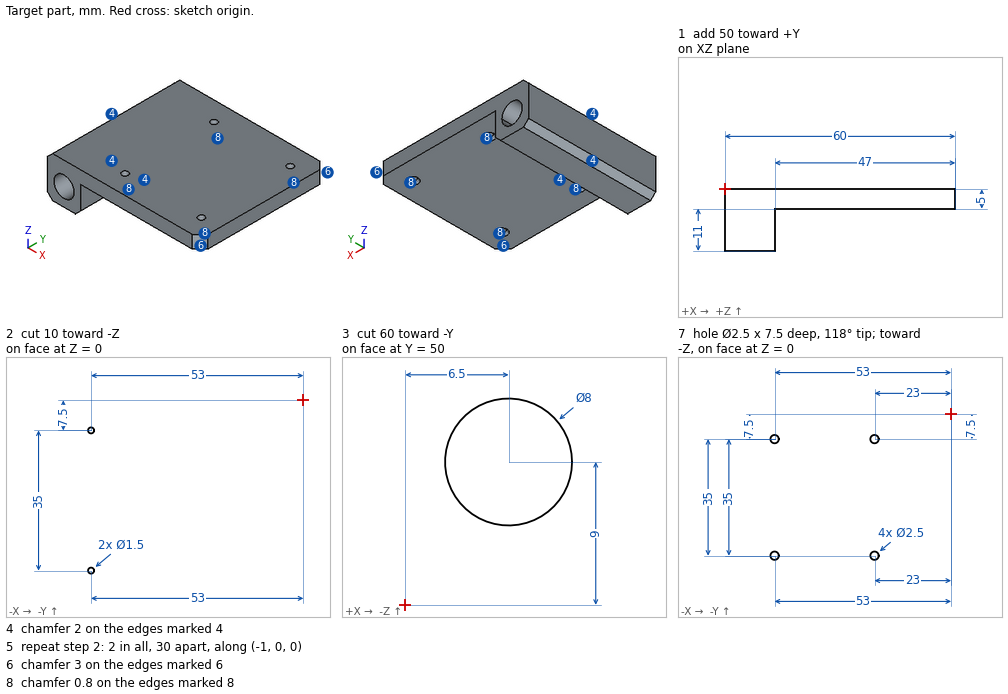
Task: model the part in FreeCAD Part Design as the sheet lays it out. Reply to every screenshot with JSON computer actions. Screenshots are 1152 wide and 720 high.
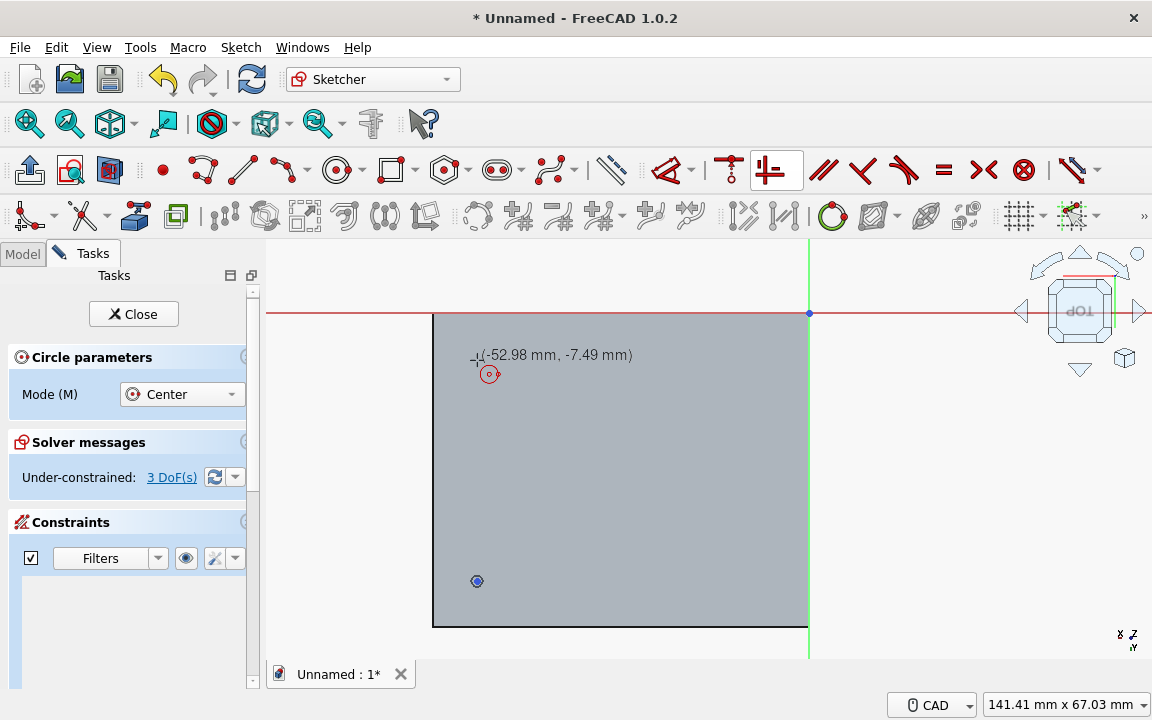
{"action": "left_click", "coordinate": [477, 360]}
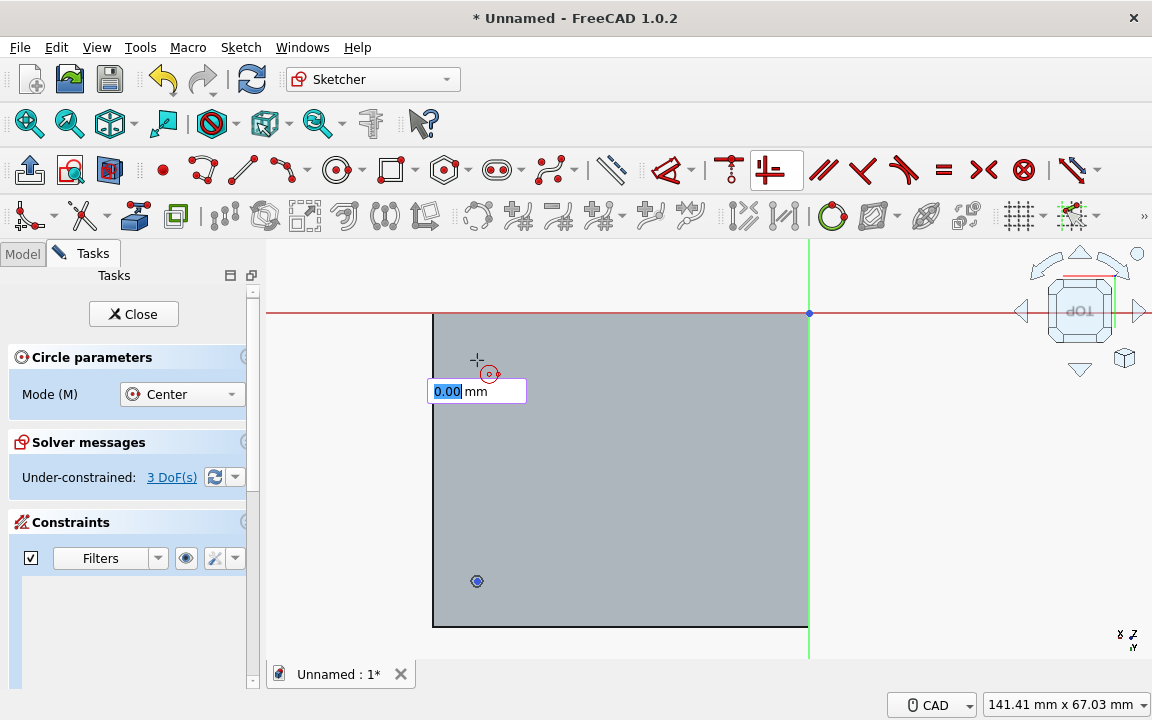
{"action": "scroll", "coordinate": [480, 357], "scroll_direction": "up", "scroll_amount": 7}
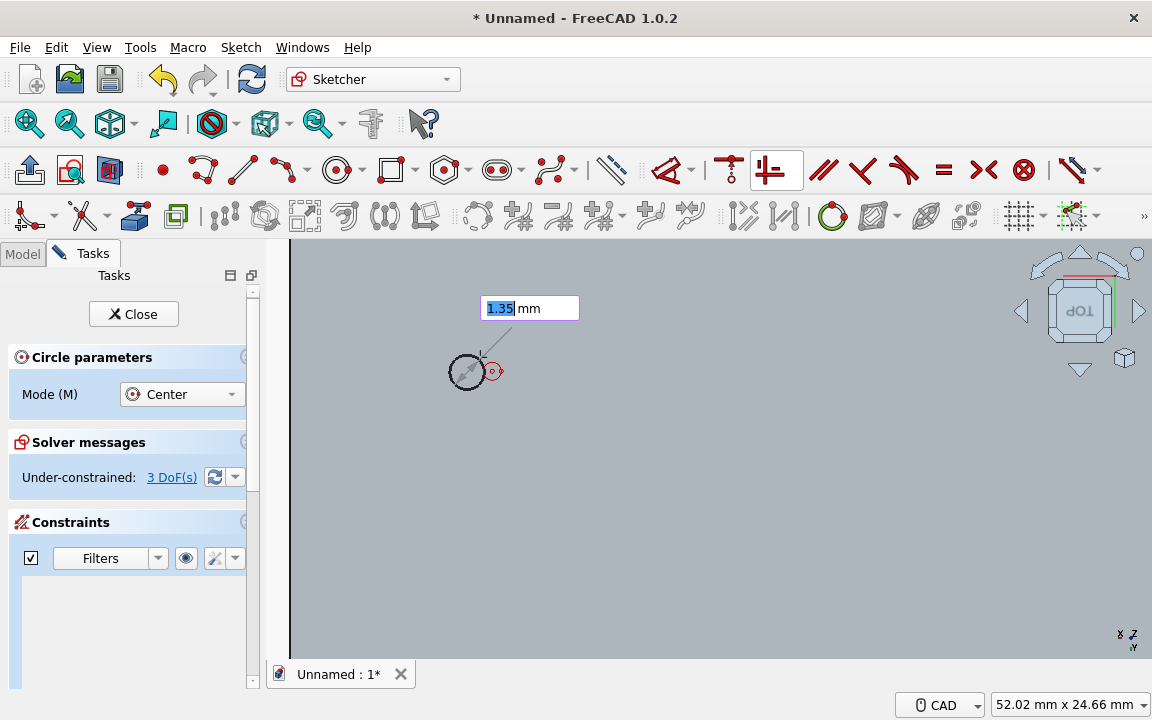
{"action": "left_click", "coordinate": [481, 357]}
{"action": "key", "text": "Escape"}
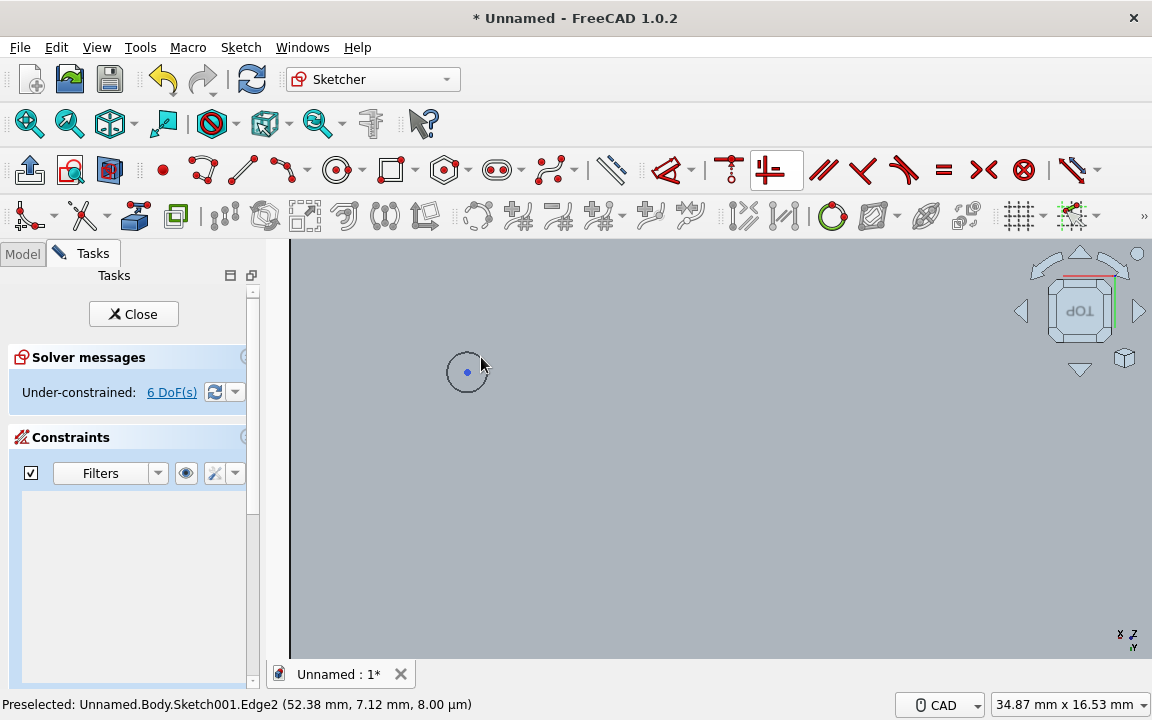
{"action": "scroll", "coordinate": [480, 357], "scroll_direction": "down", "scroll_amount": 7}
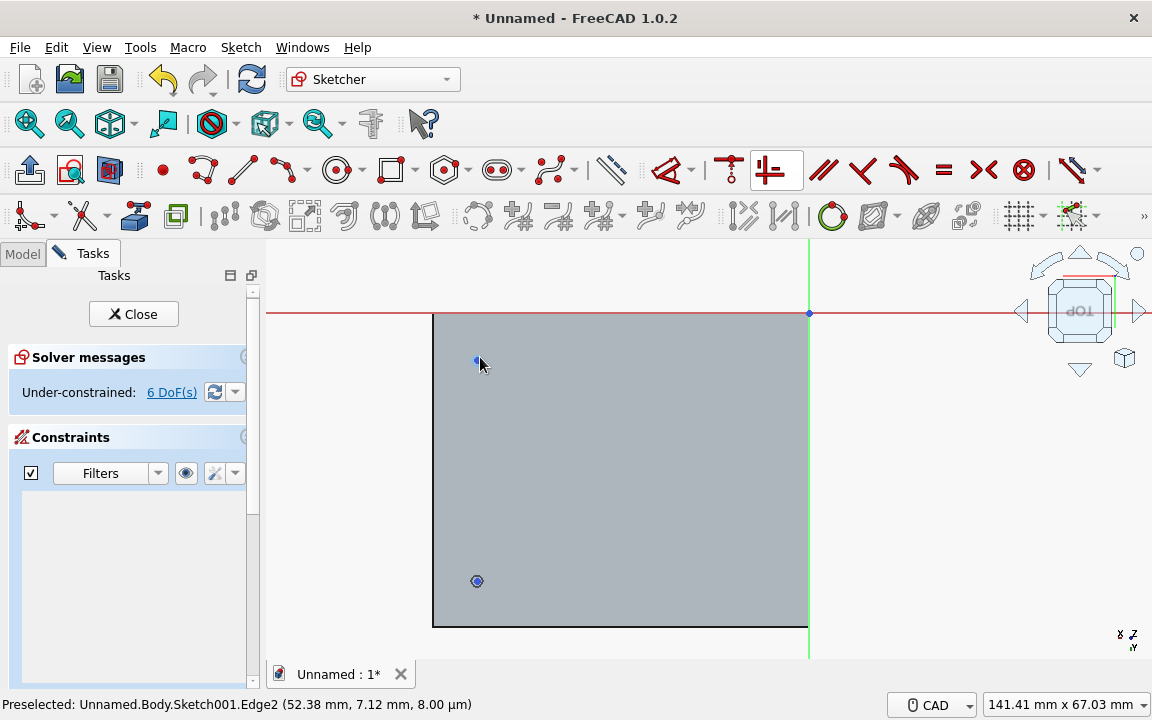
{"action": "scroll", "coordinate": [481, 577], "scroll_direction": "up", "scroll_amount": 5}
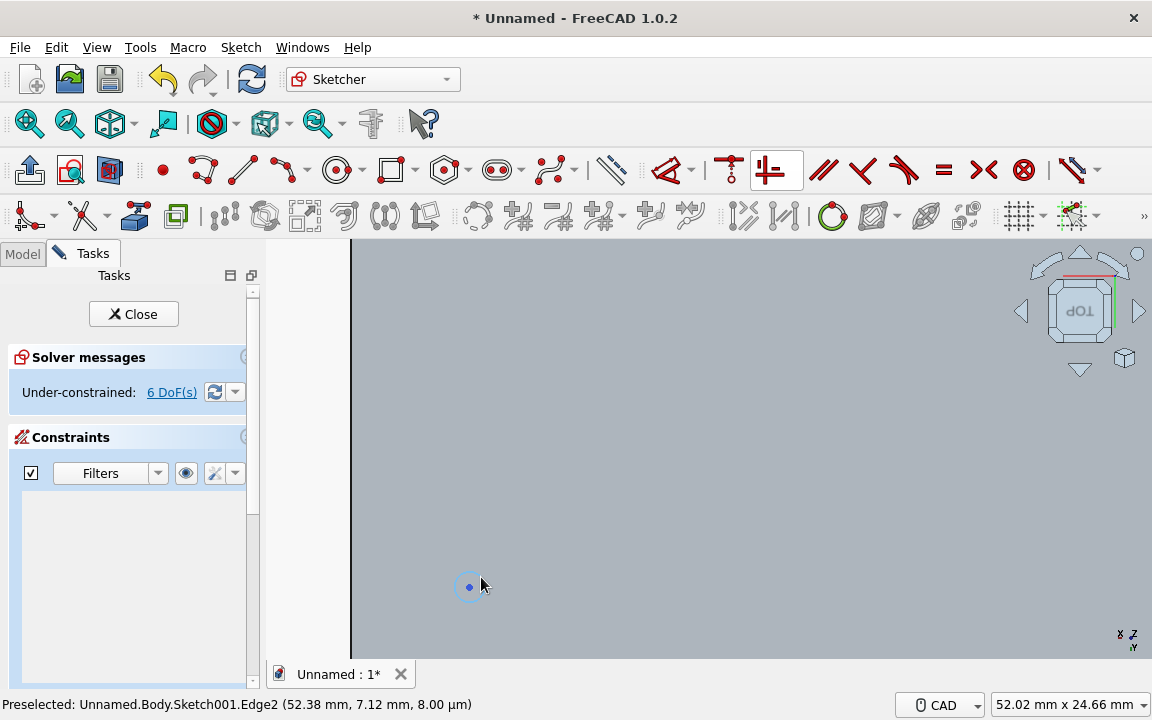
{"action": "left_click", "coordinate": [480, 576]}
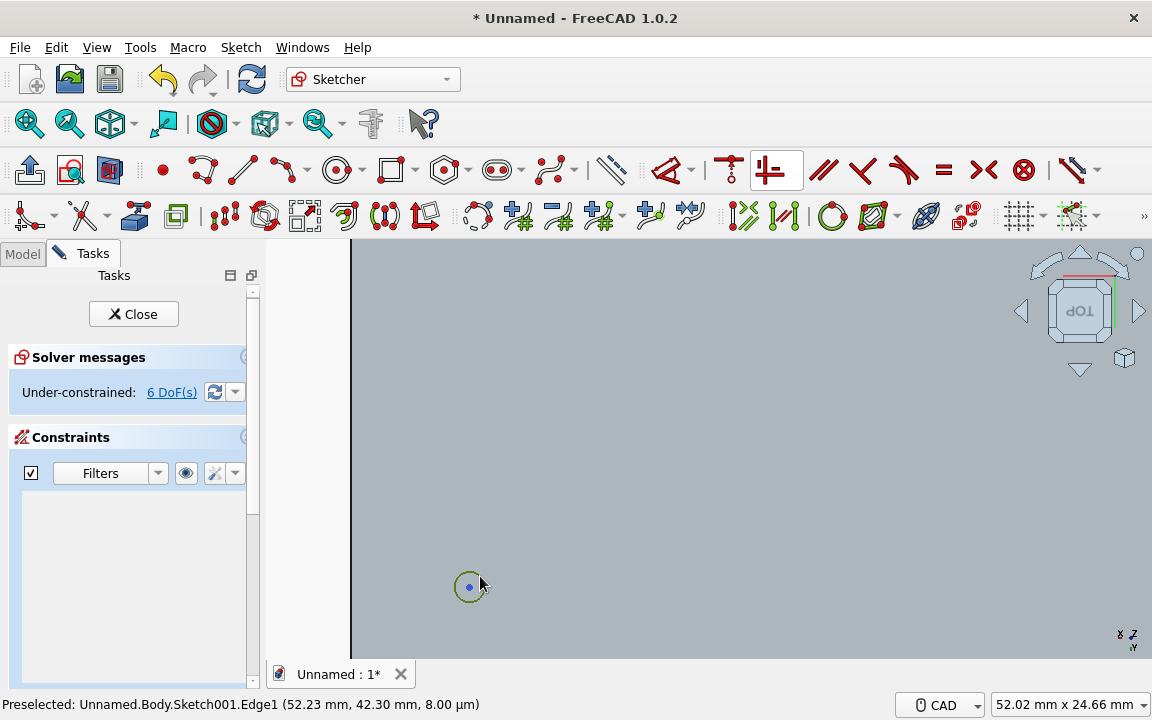
{"action": "scroll", "coordinate": [481, 578], "scroll_direction": "down", "scroll_amount": 5}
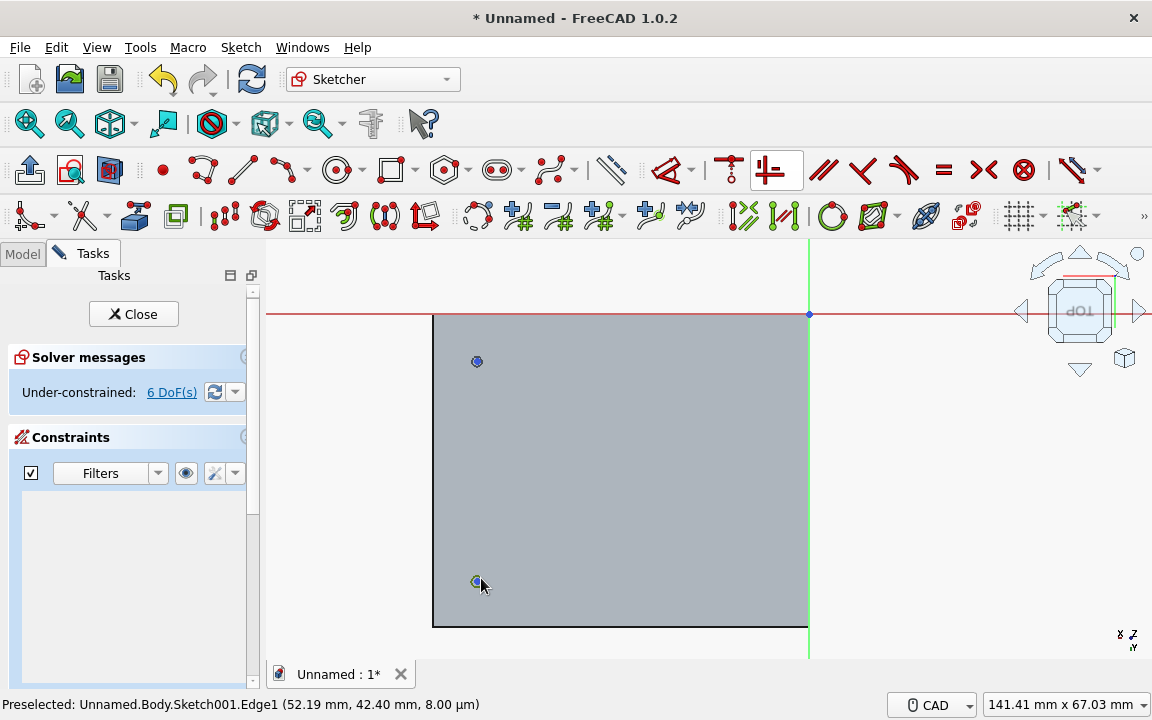
{"action": "scroll", "coordinate": [480, 358], "scroll_direction": "up", "scroll_amount": 6}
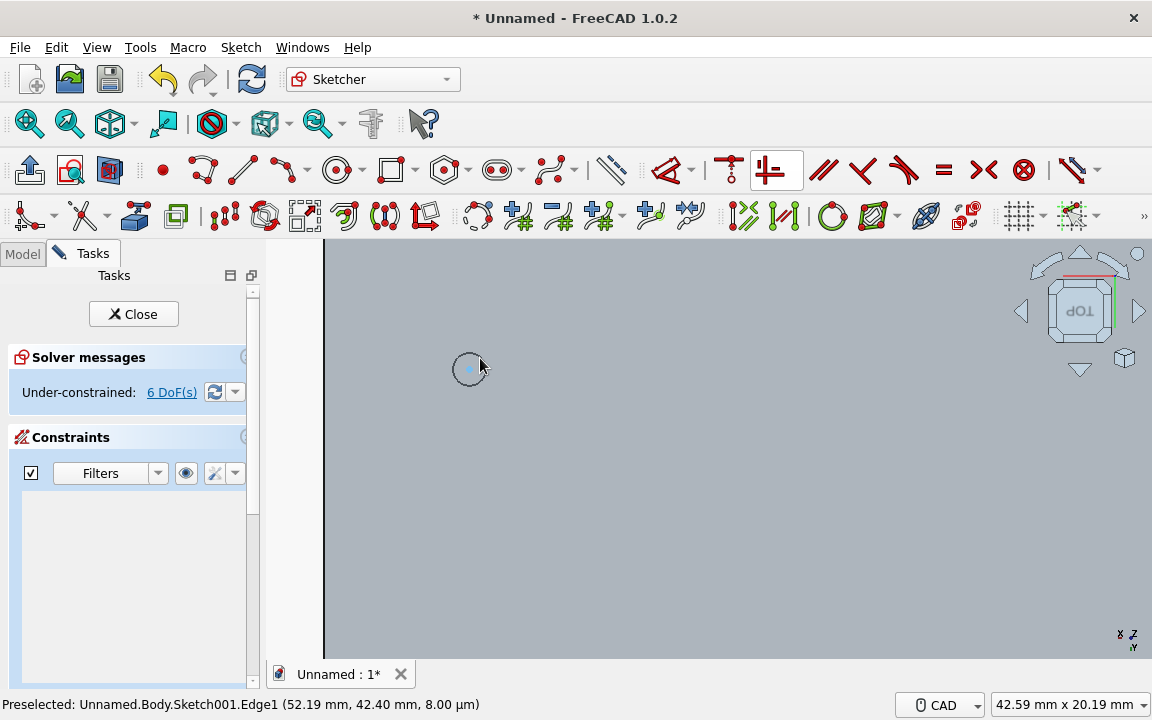
{"action": "left_click", "coordinate": [481, 358]}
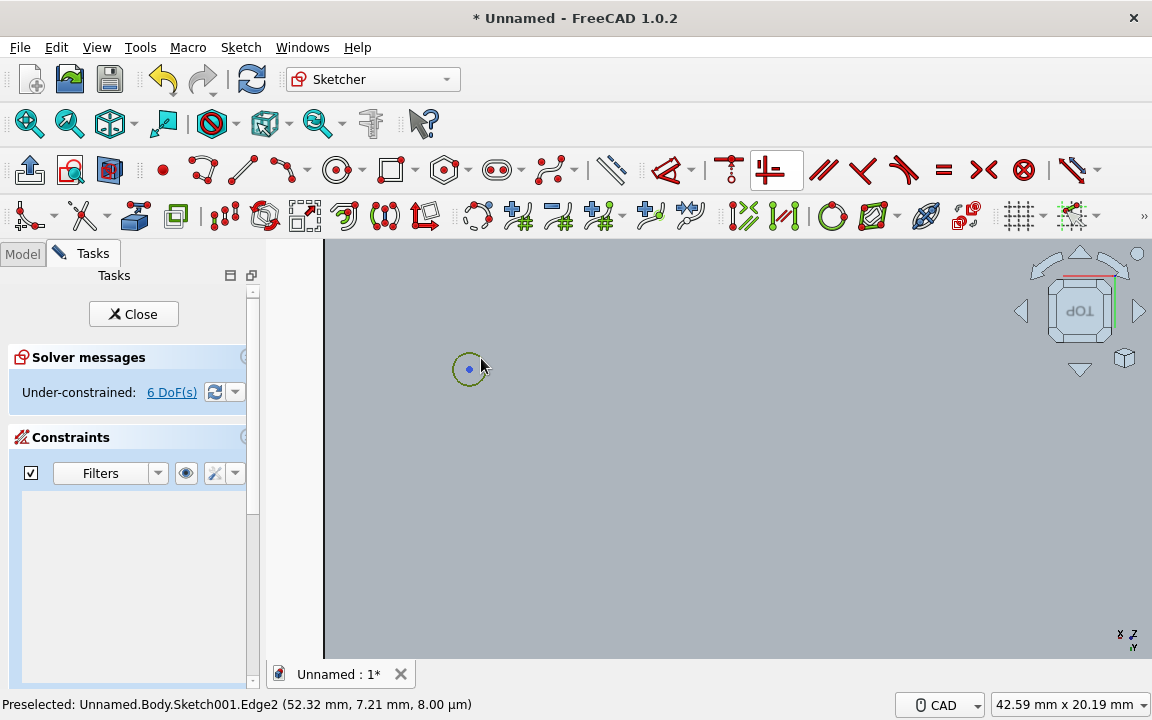
{"action": "left_click", "coordinate": [944, 170]}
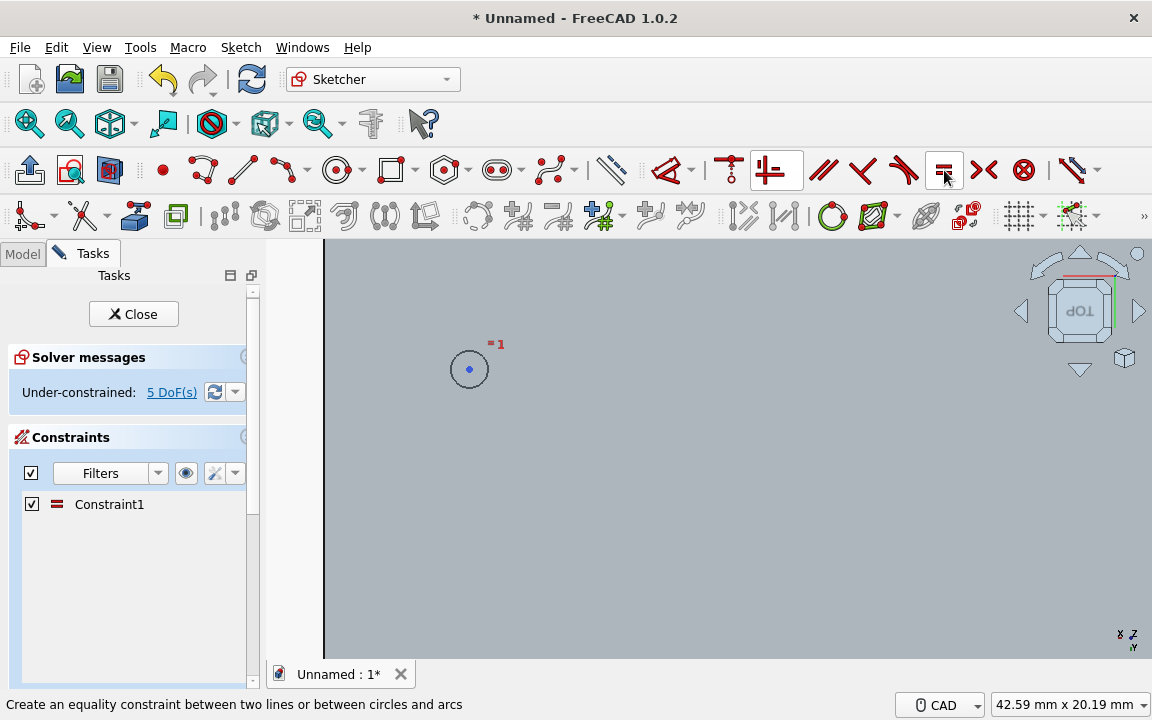
{"action": "key", "text": "d"}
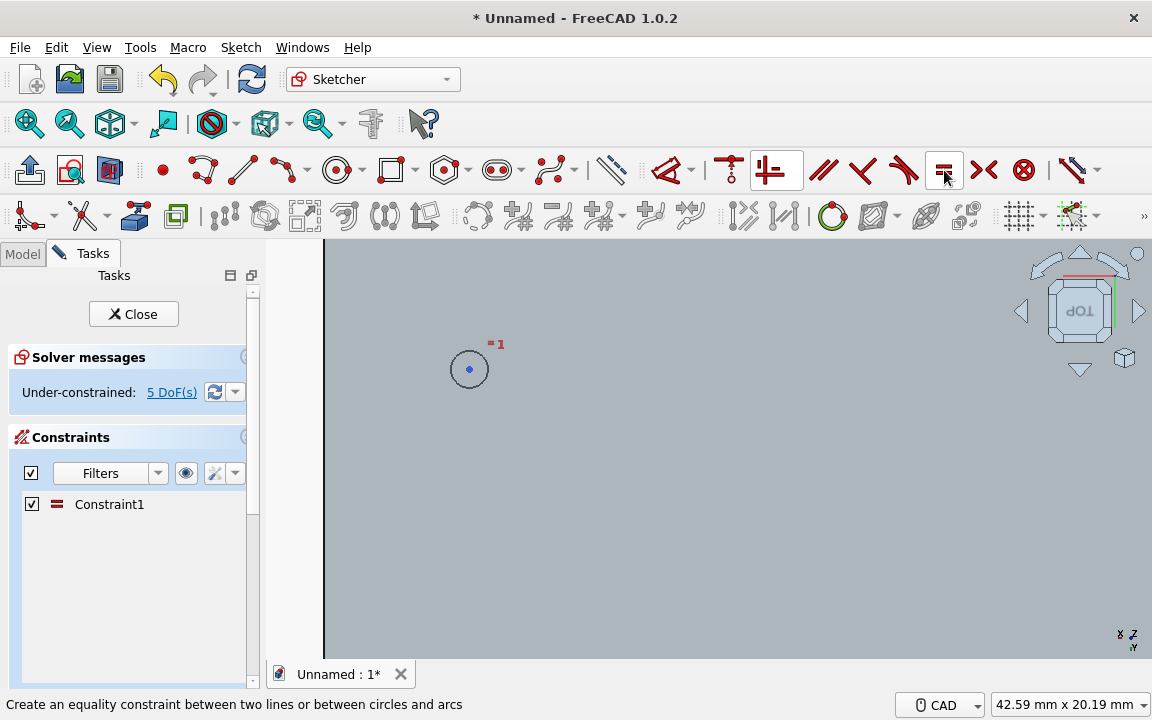
{"action": "scroll", "coordinate": [480, 357], "scroll_direction": "down", "scroll_amount": 6}